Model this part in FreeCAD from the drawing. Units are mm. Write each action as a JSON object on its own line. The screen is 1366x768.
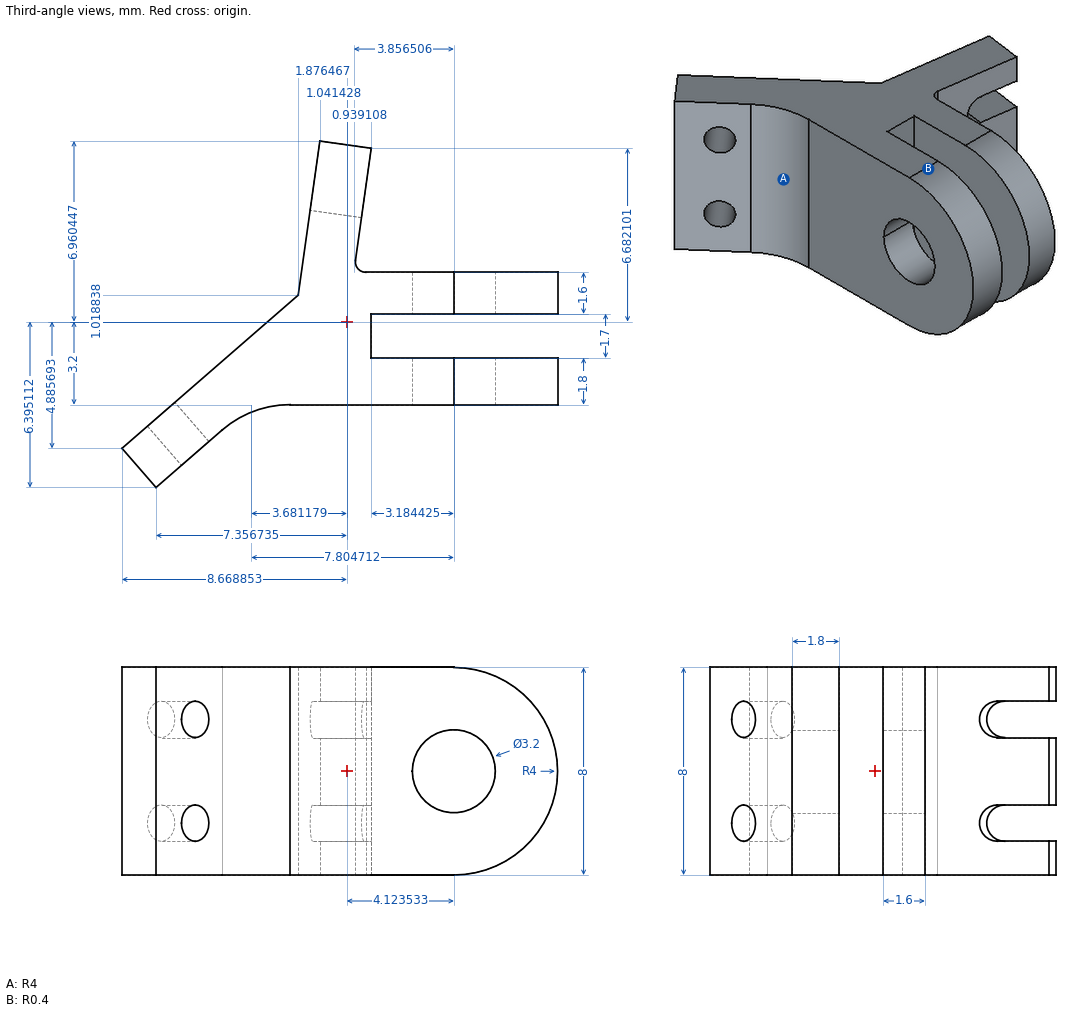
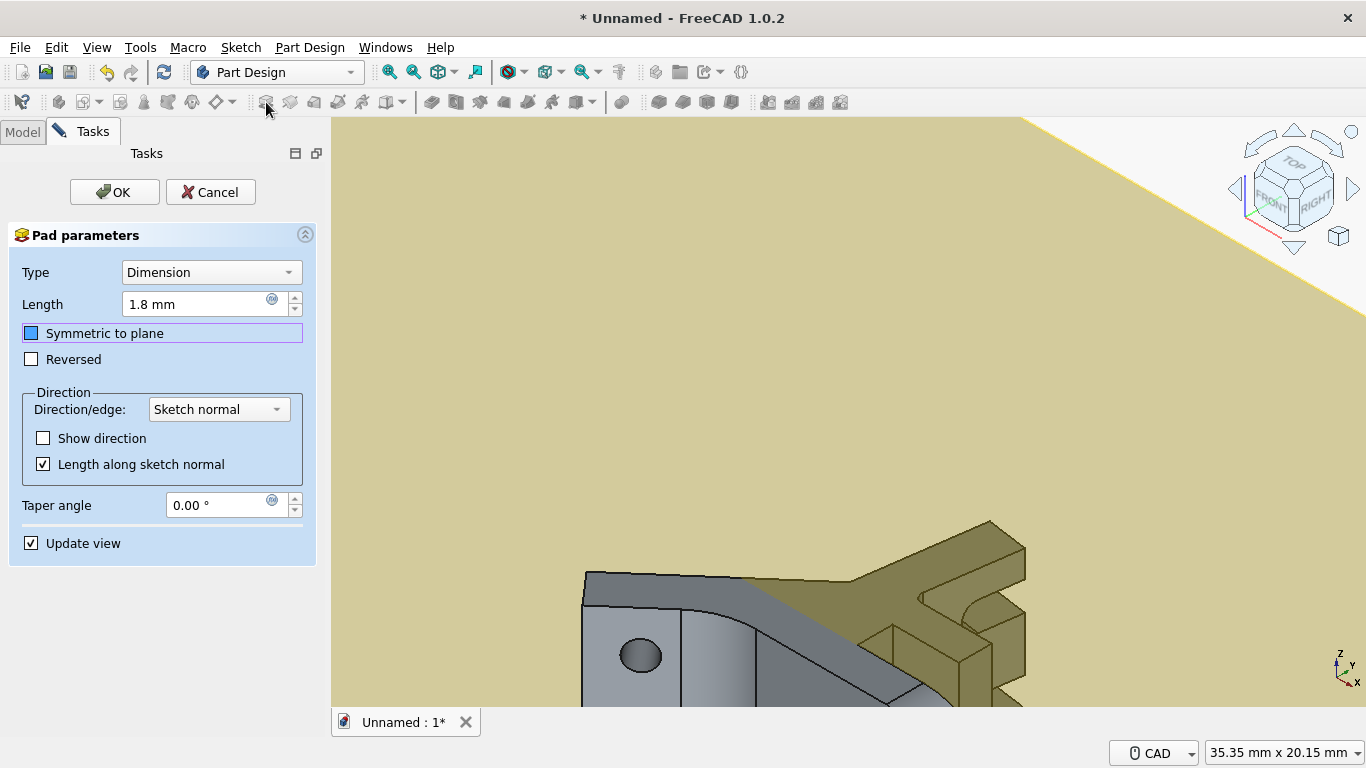
{"action": "left_click", "coordinate": [115, 192]}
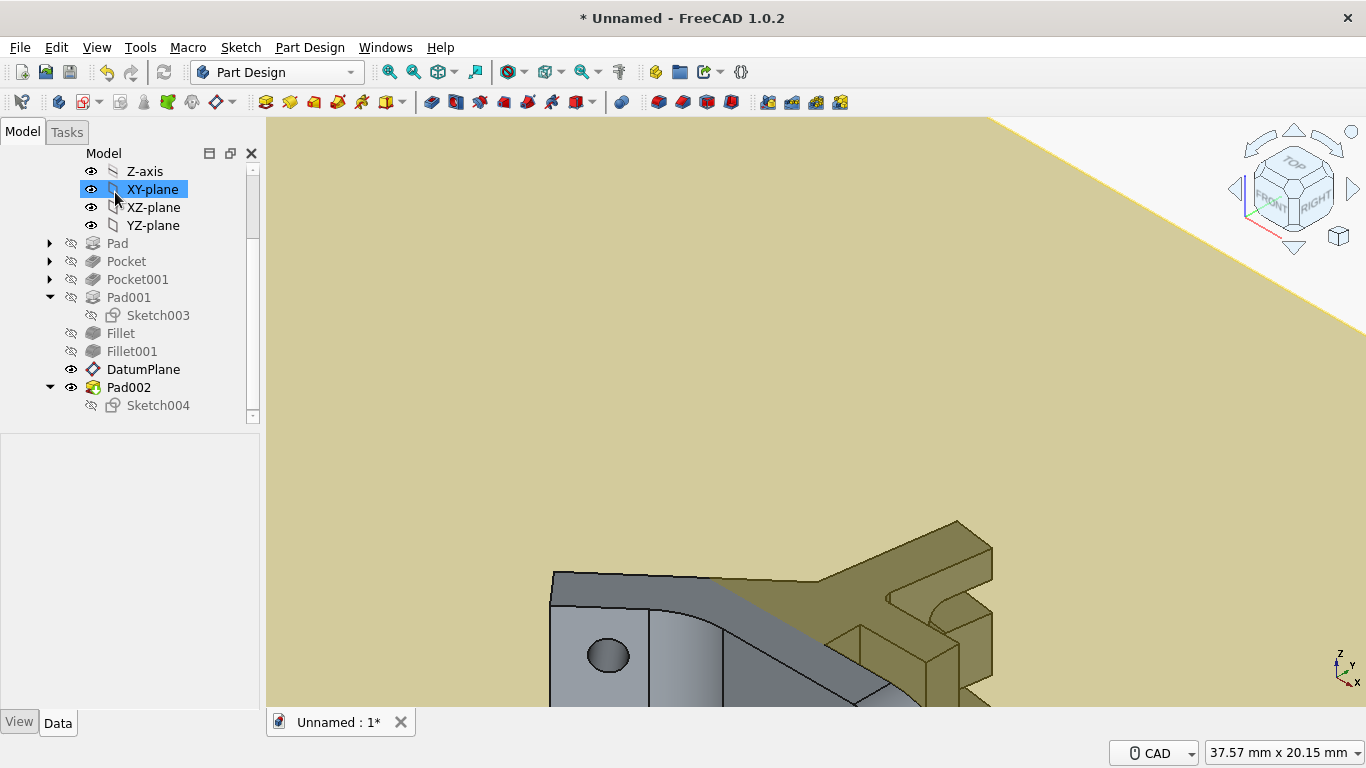
{"action": "left_click", "coordinate": [116, 369]}
{"action": "key", "text": "space"}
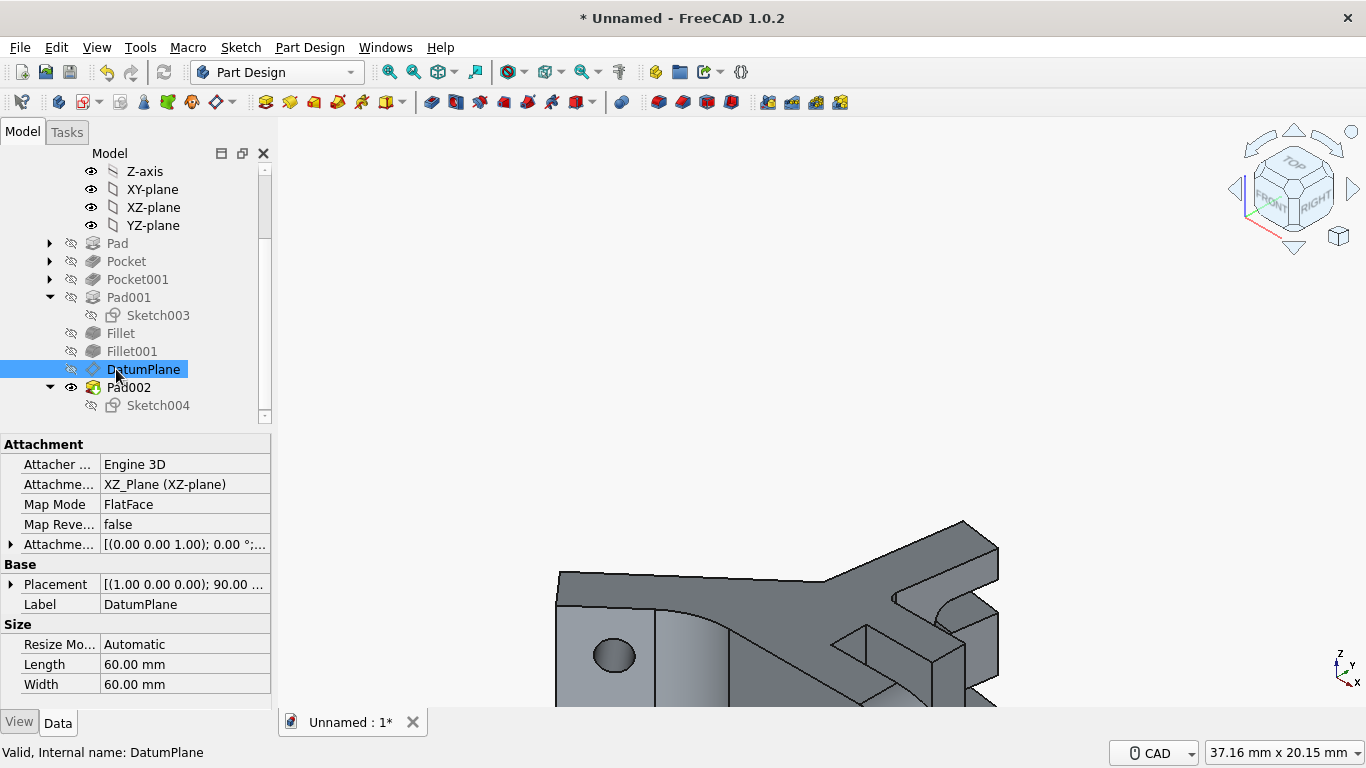
{"action": "left_click", "coordinate": [390, 72]}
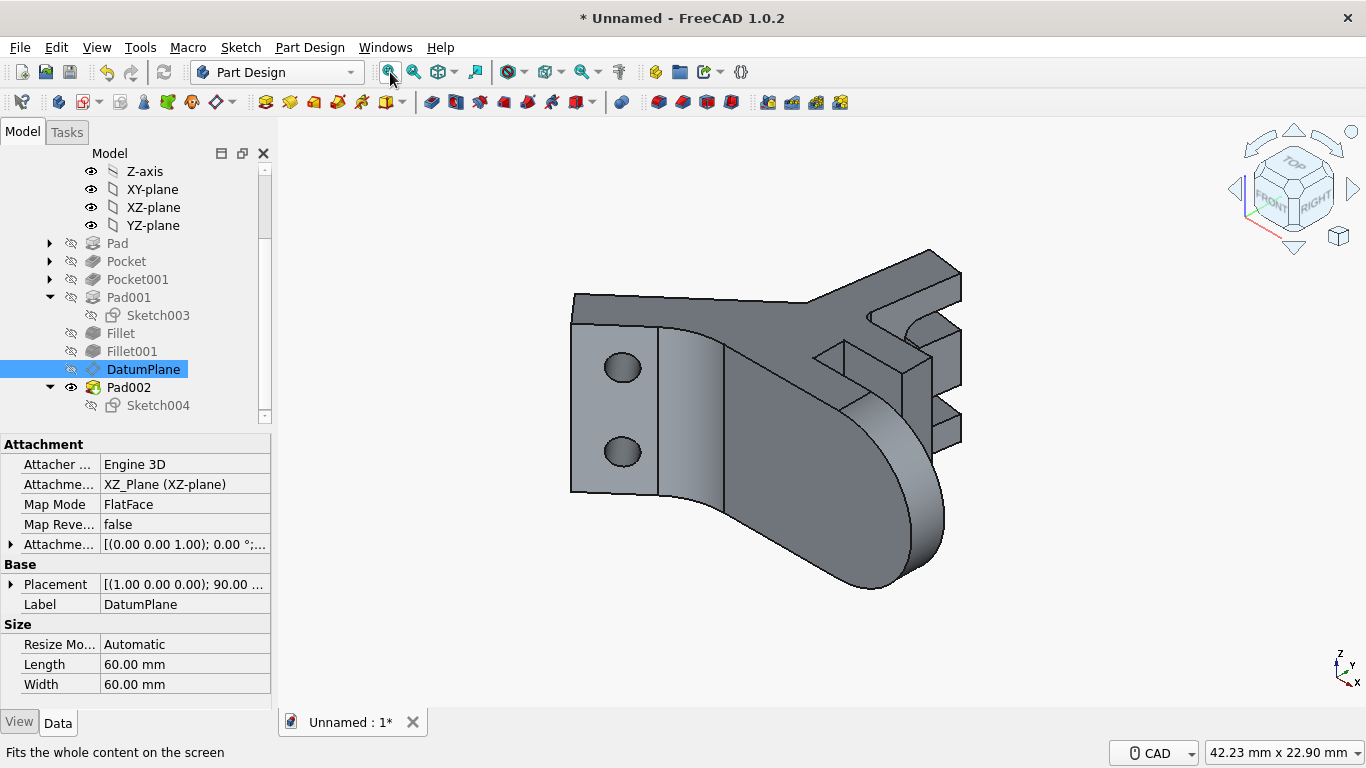
{"action": "key", "text": "4"}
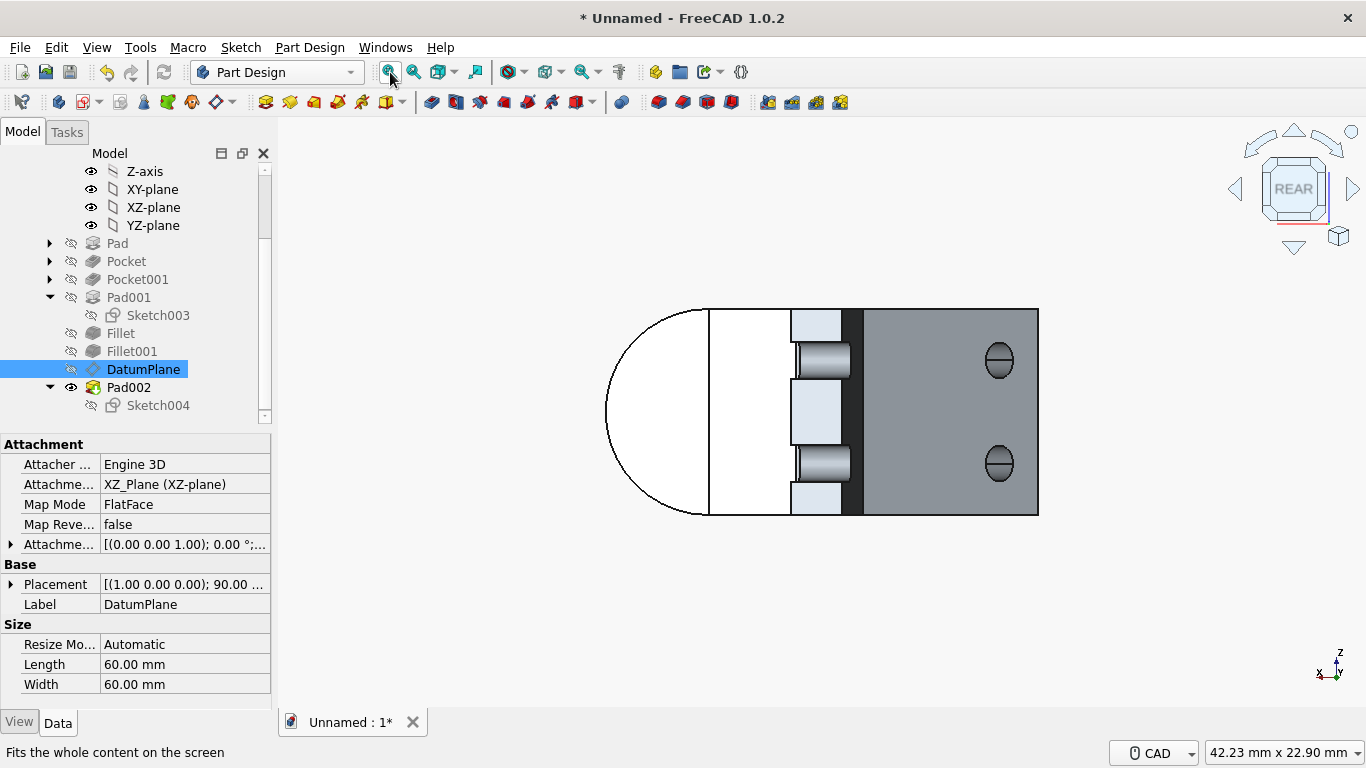
{"action": "left_click", "coordinate": [390, 72]}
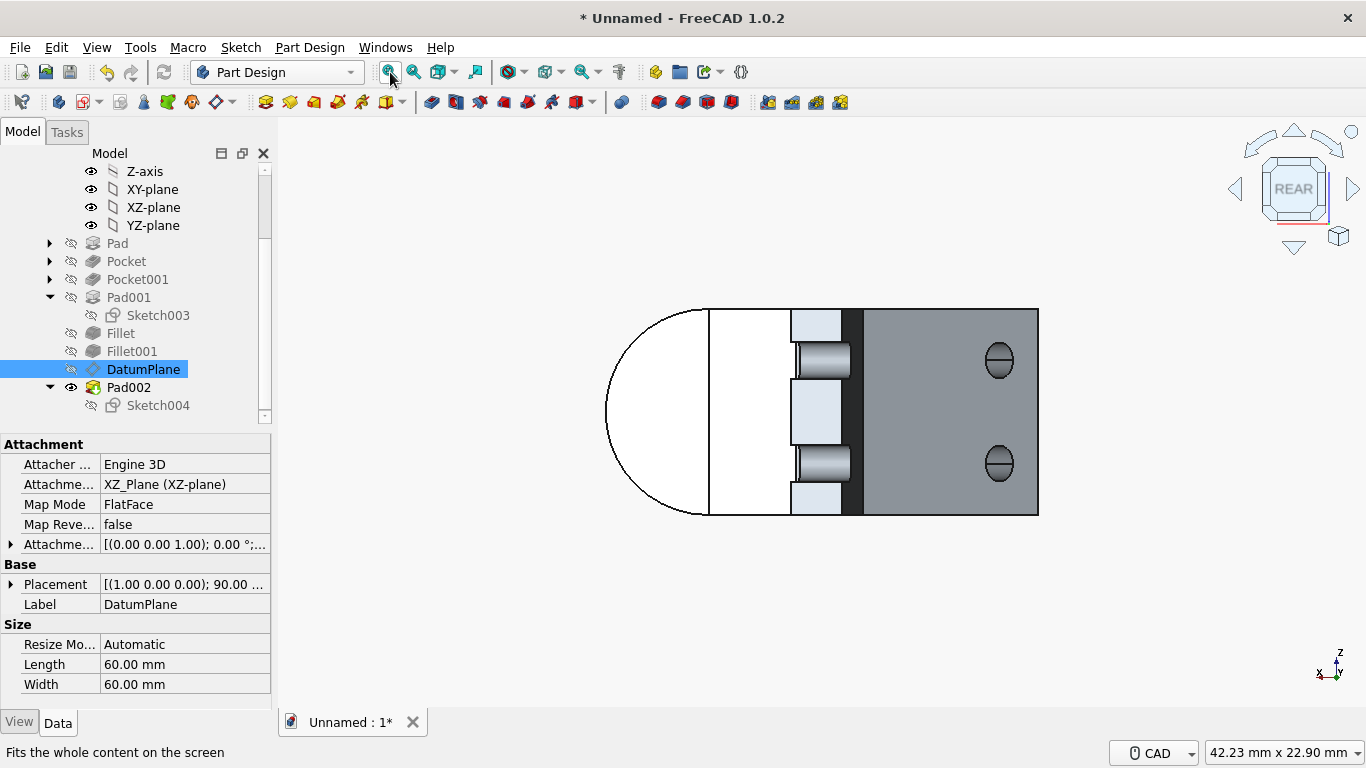
{"action": "left_click", "coordinate": [752, 352]}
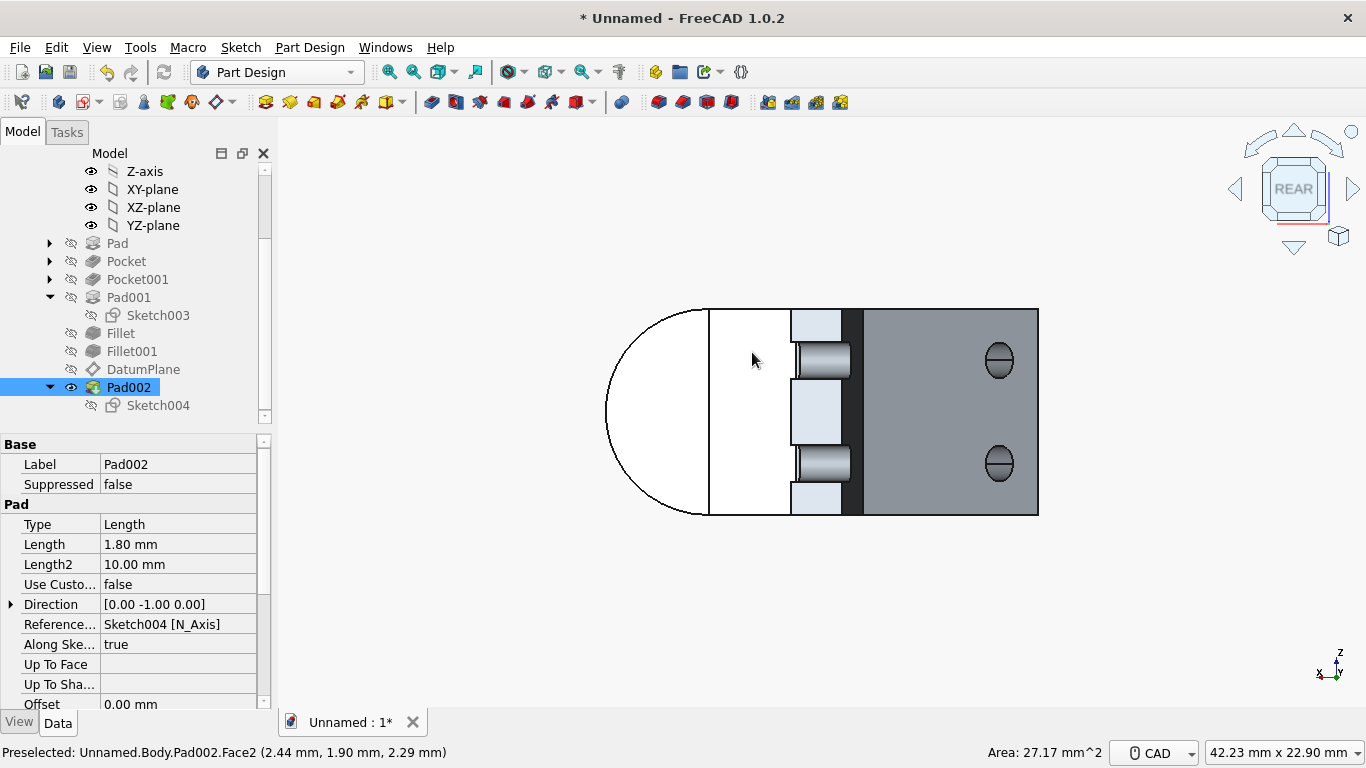
{"action": "left_click", "coordinate": [84, 102]}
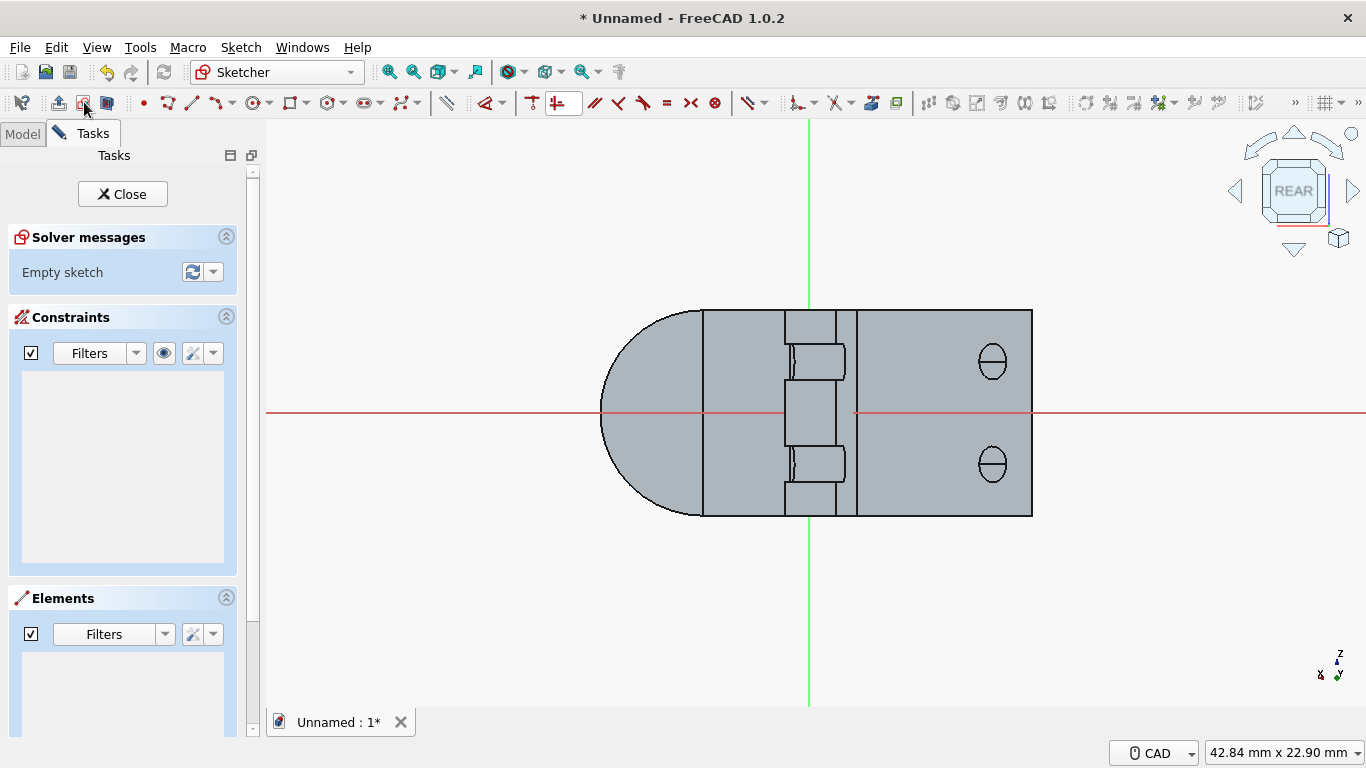
{"action": "scroll", "coordinate": [653, 413], "scroll_direction": "up", "scroll_amount": 3}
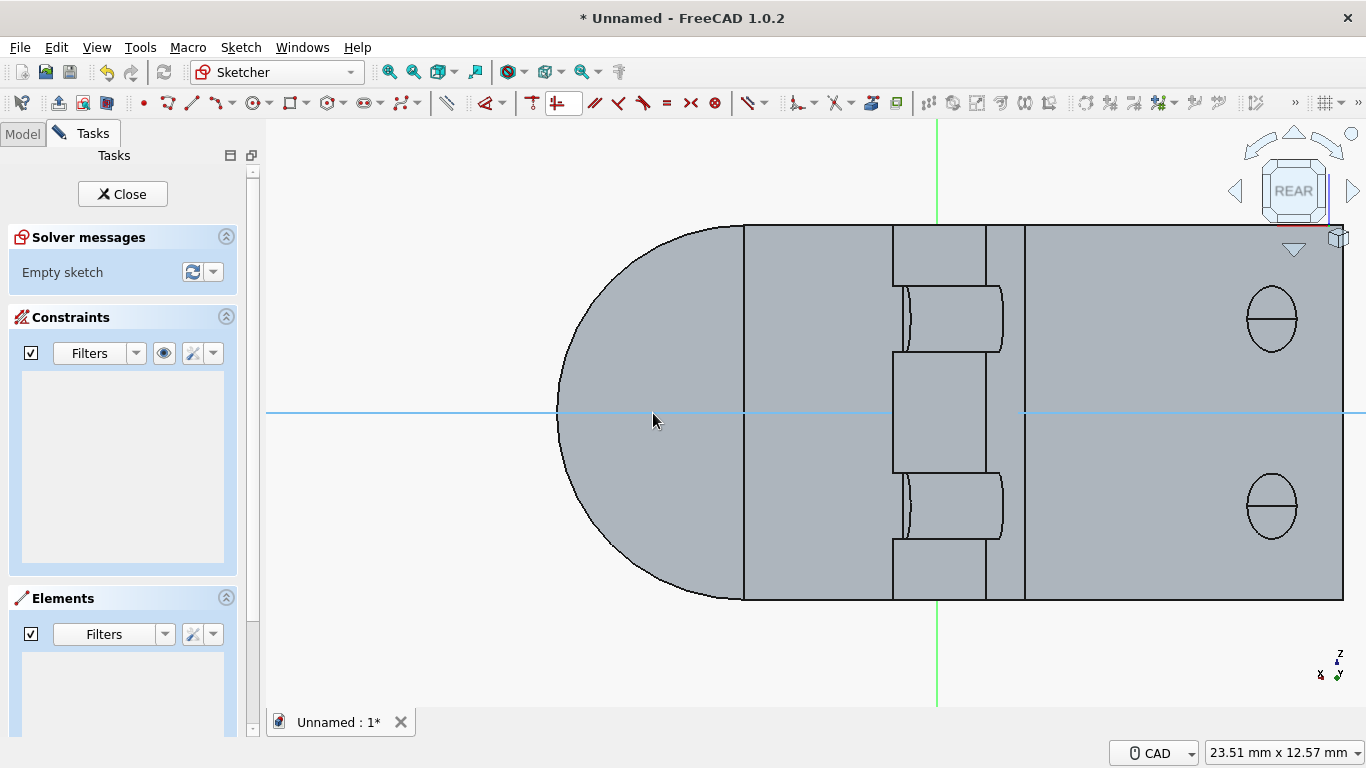
{"action": "left_click", "coordinate": [192, 104]}